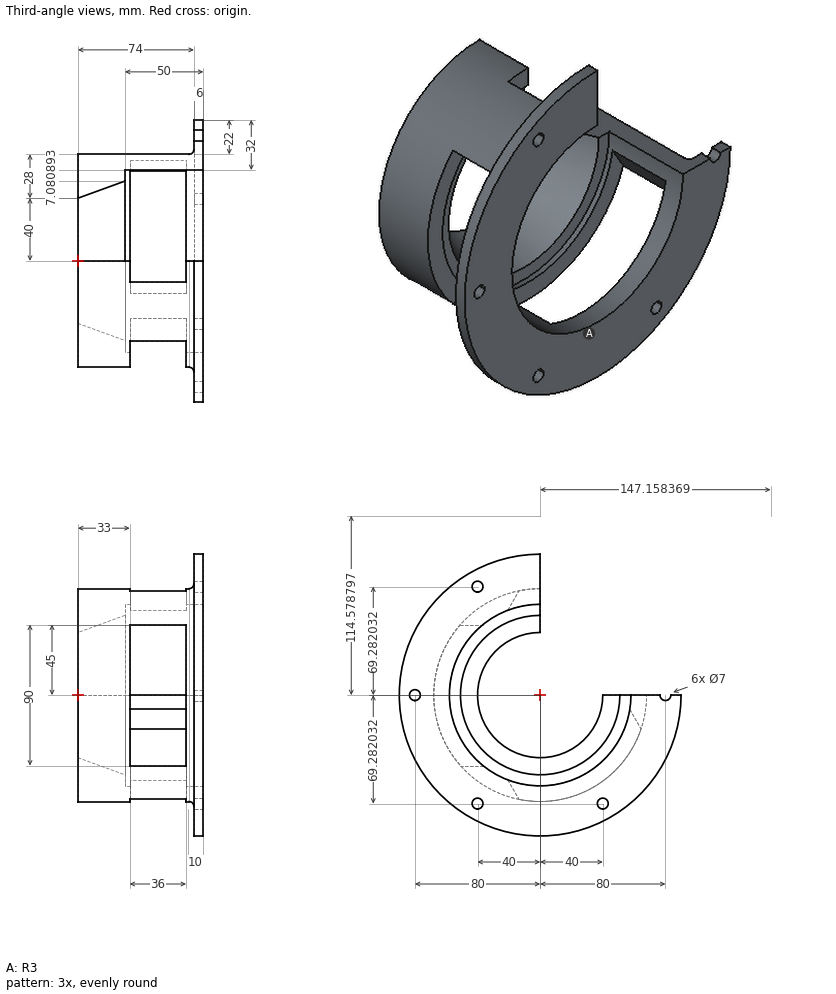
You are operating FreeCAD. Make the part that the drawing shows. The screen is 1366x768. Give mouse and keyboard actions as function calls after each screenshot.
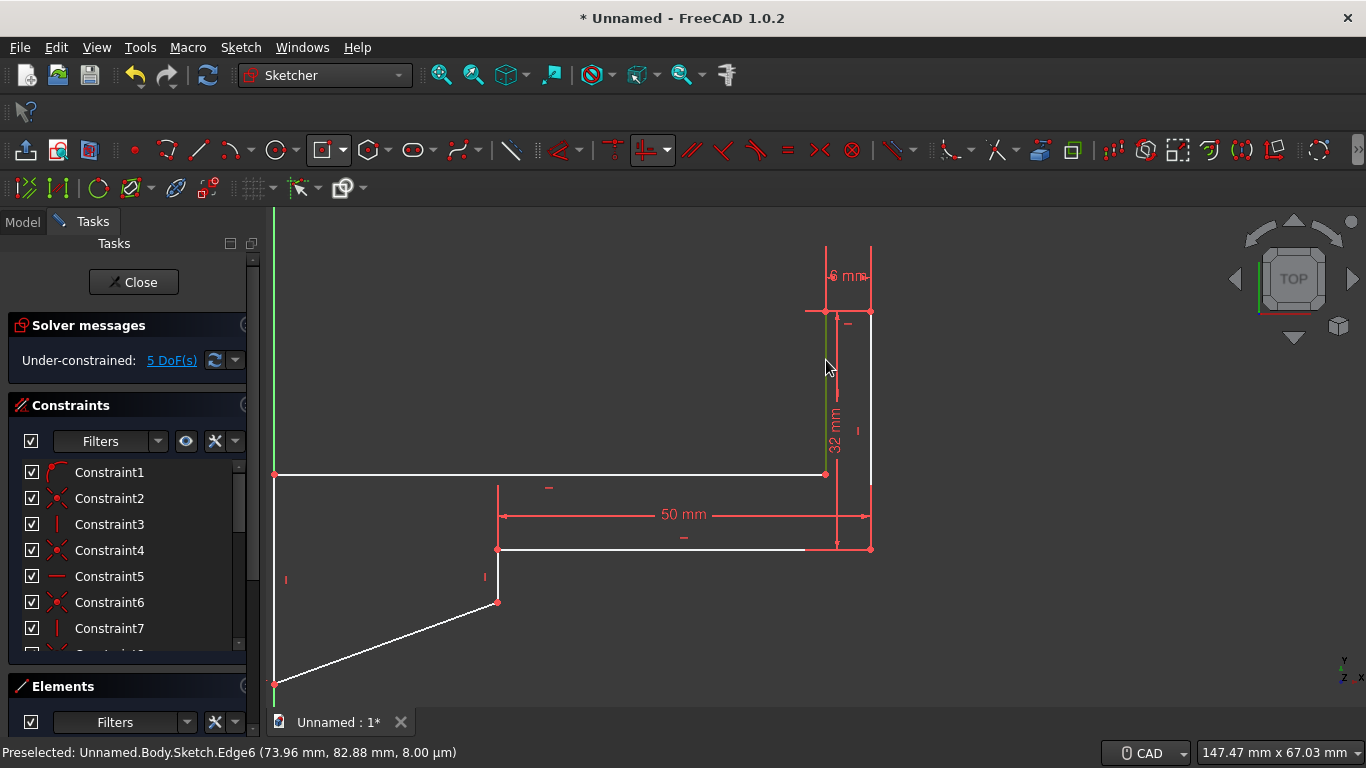
key(i)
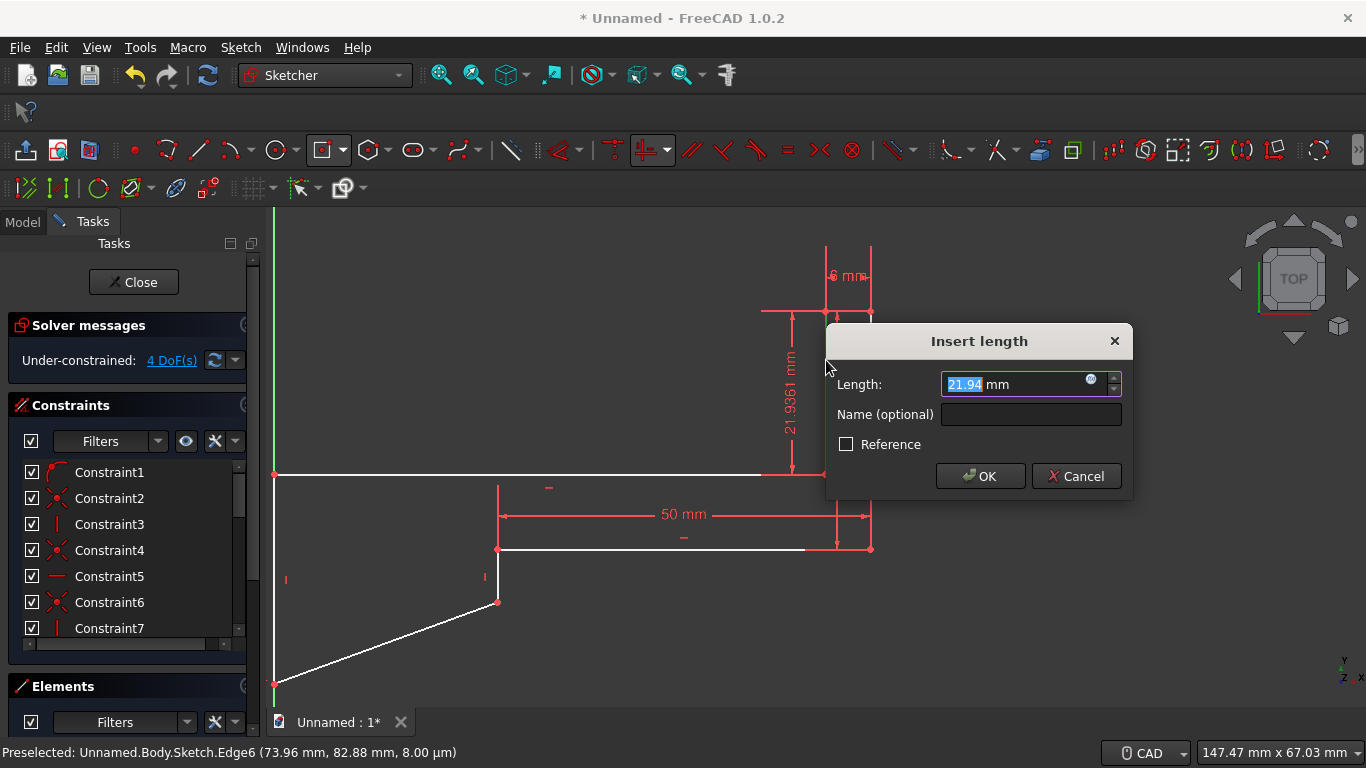
text(22)
key(Return)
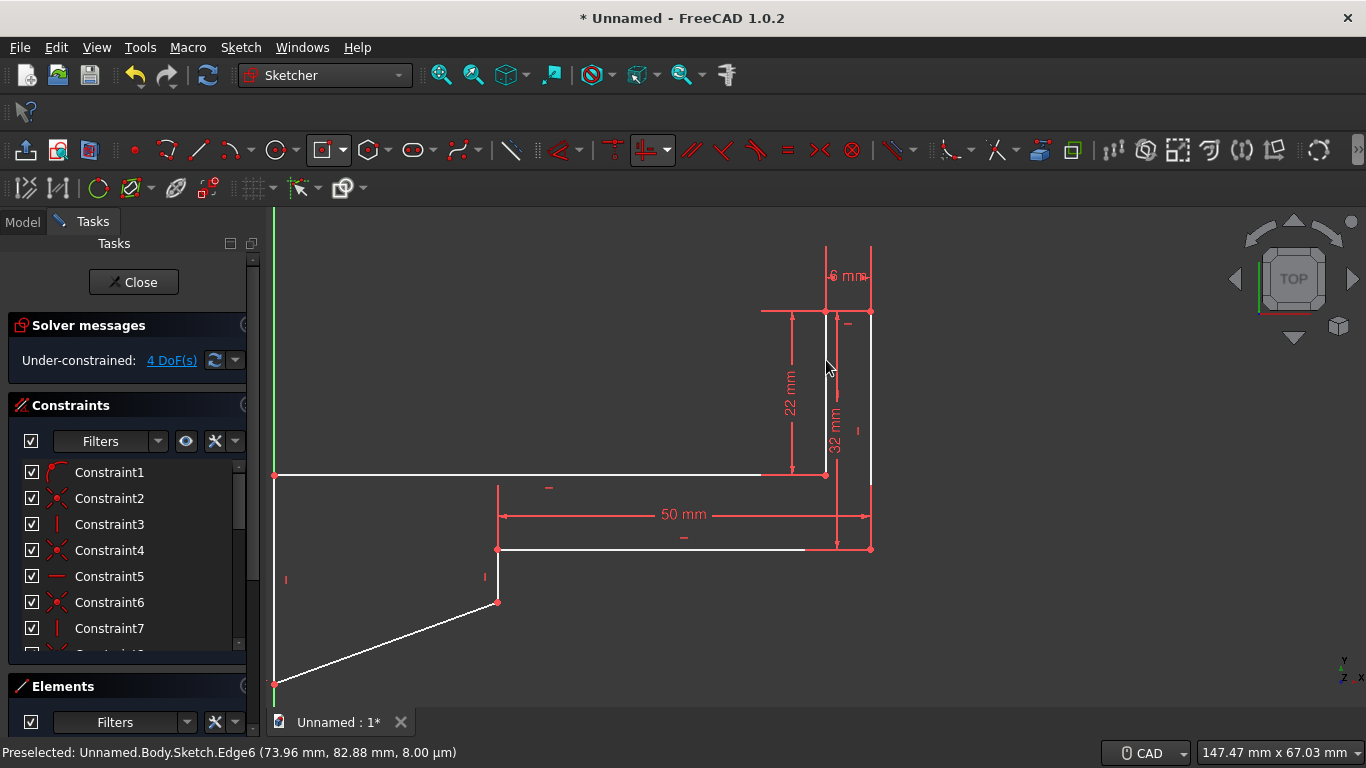
click(660, 475)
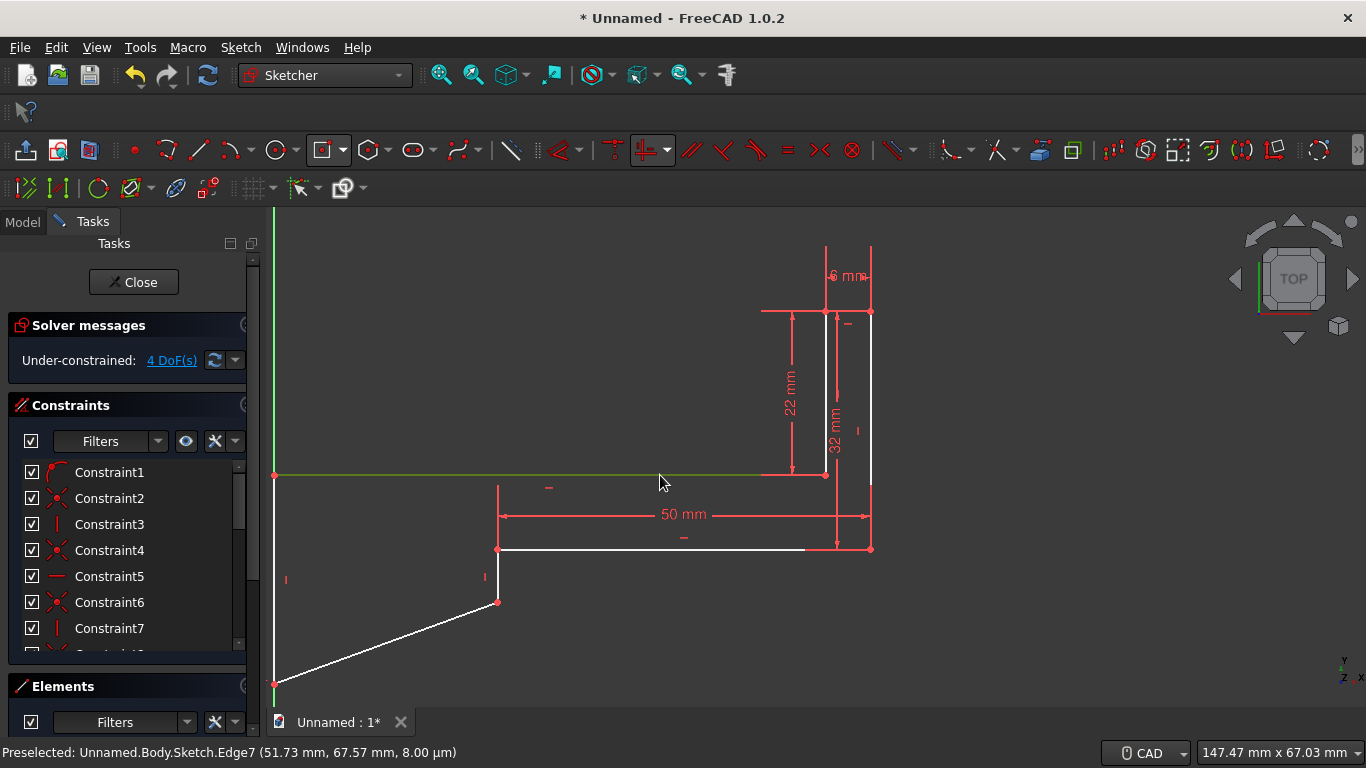
click(582, 150)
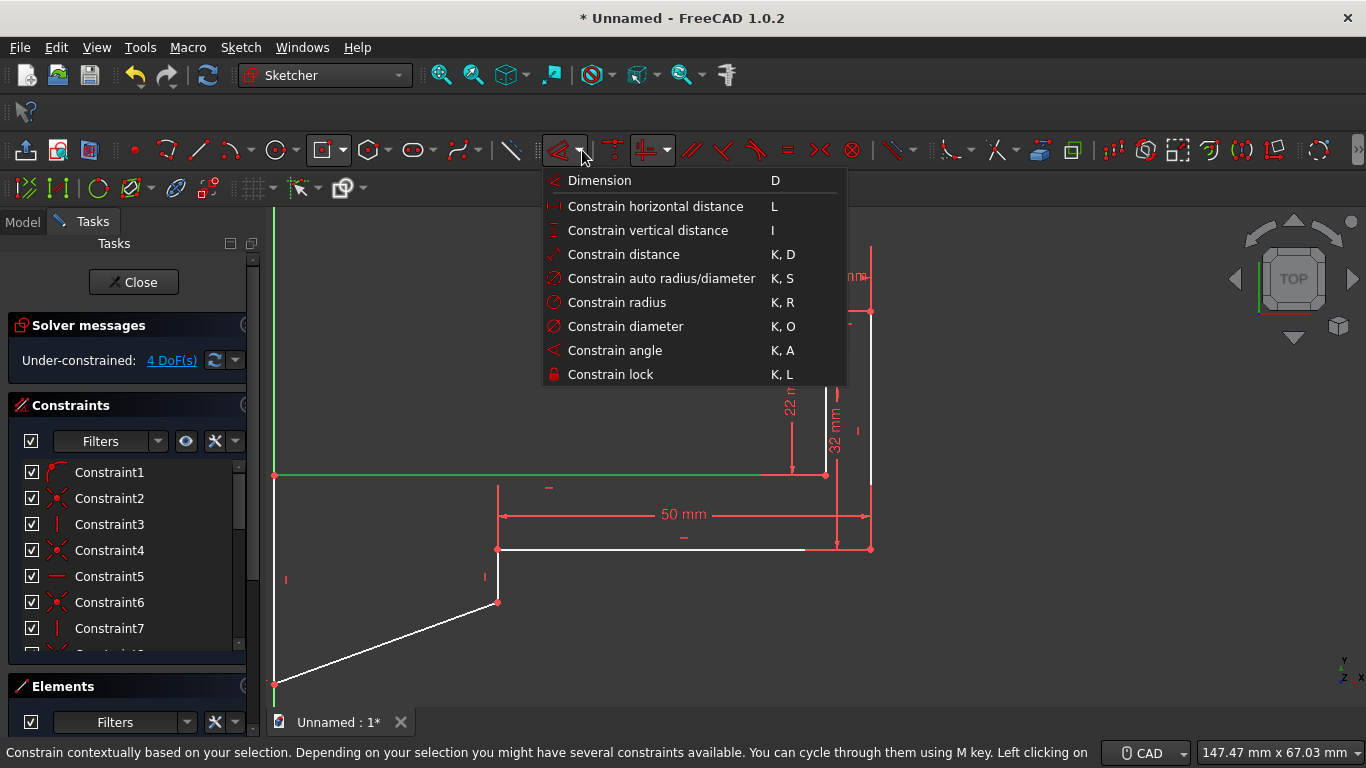
click(695, 206)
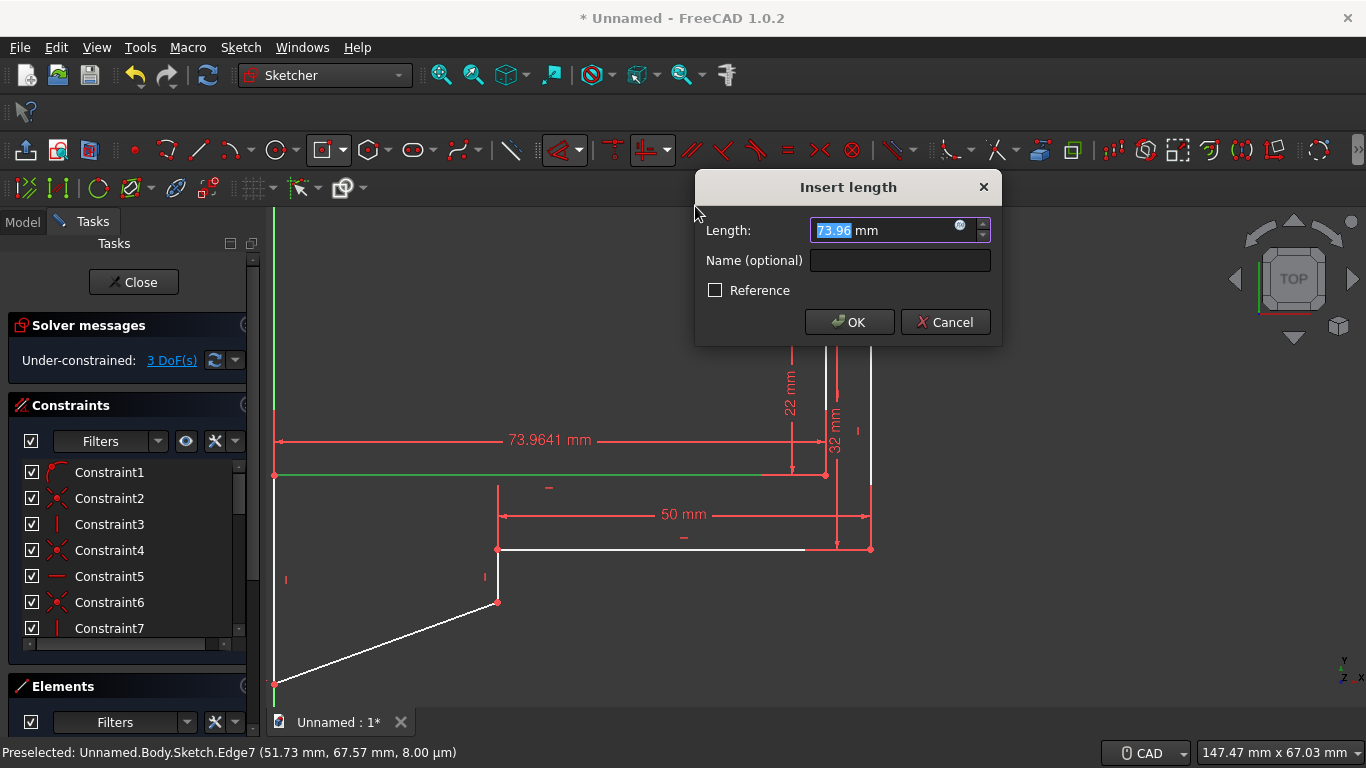
text(74)
key(Return)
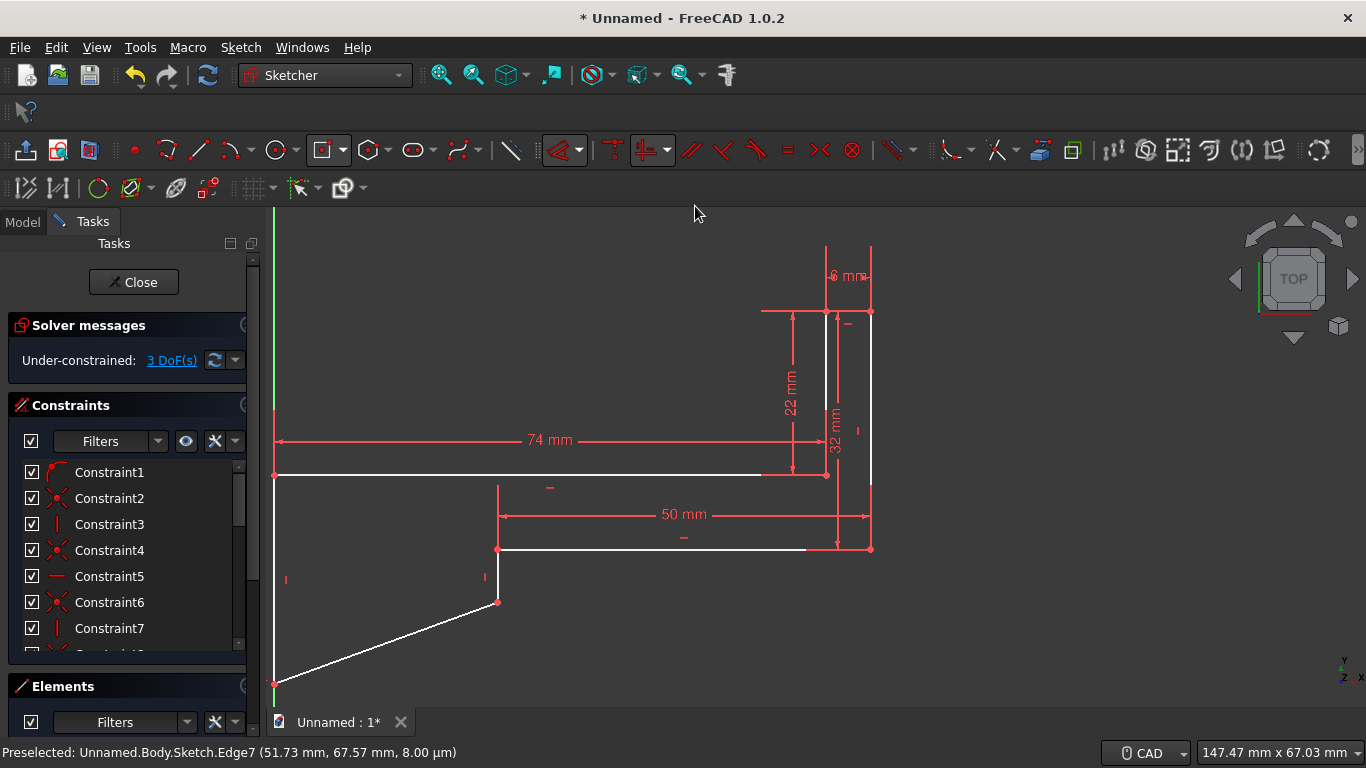
scroll(890, 305, down, 4)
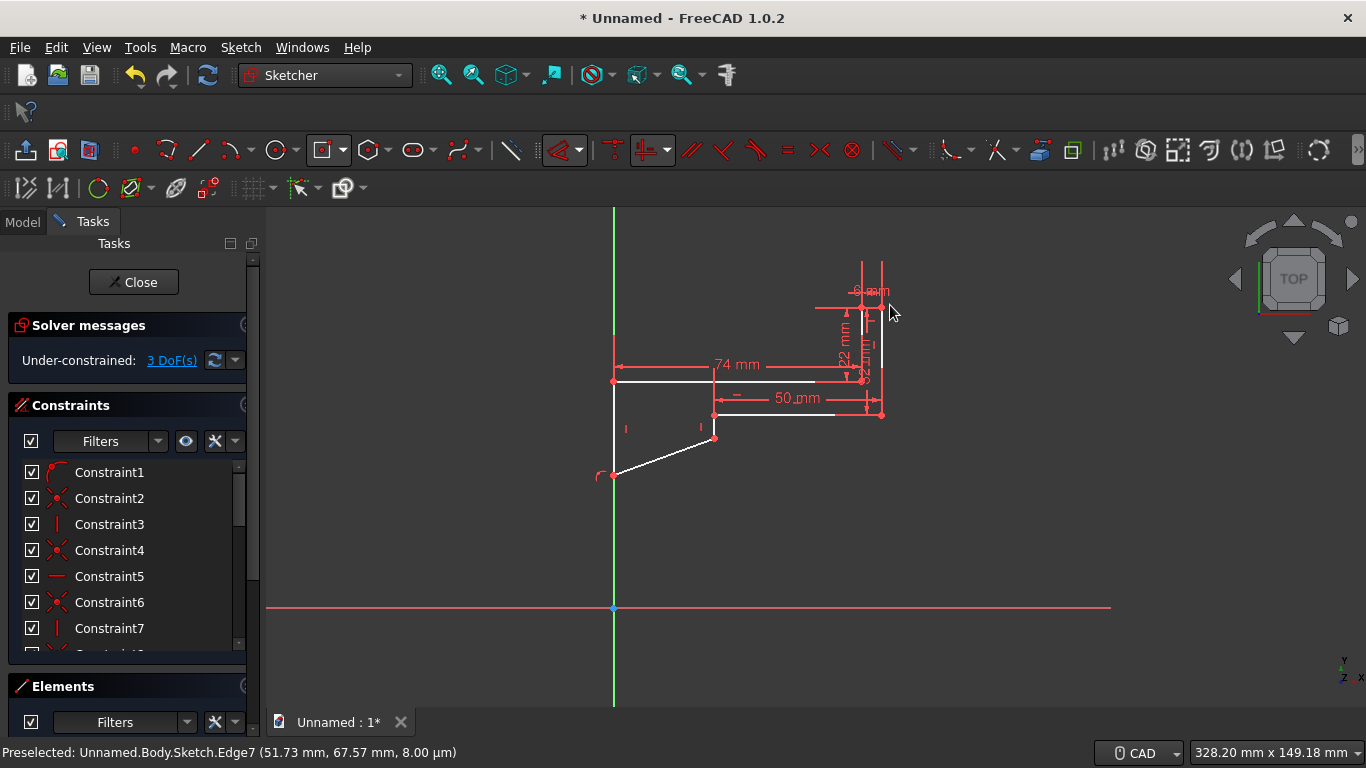
click(614, 410)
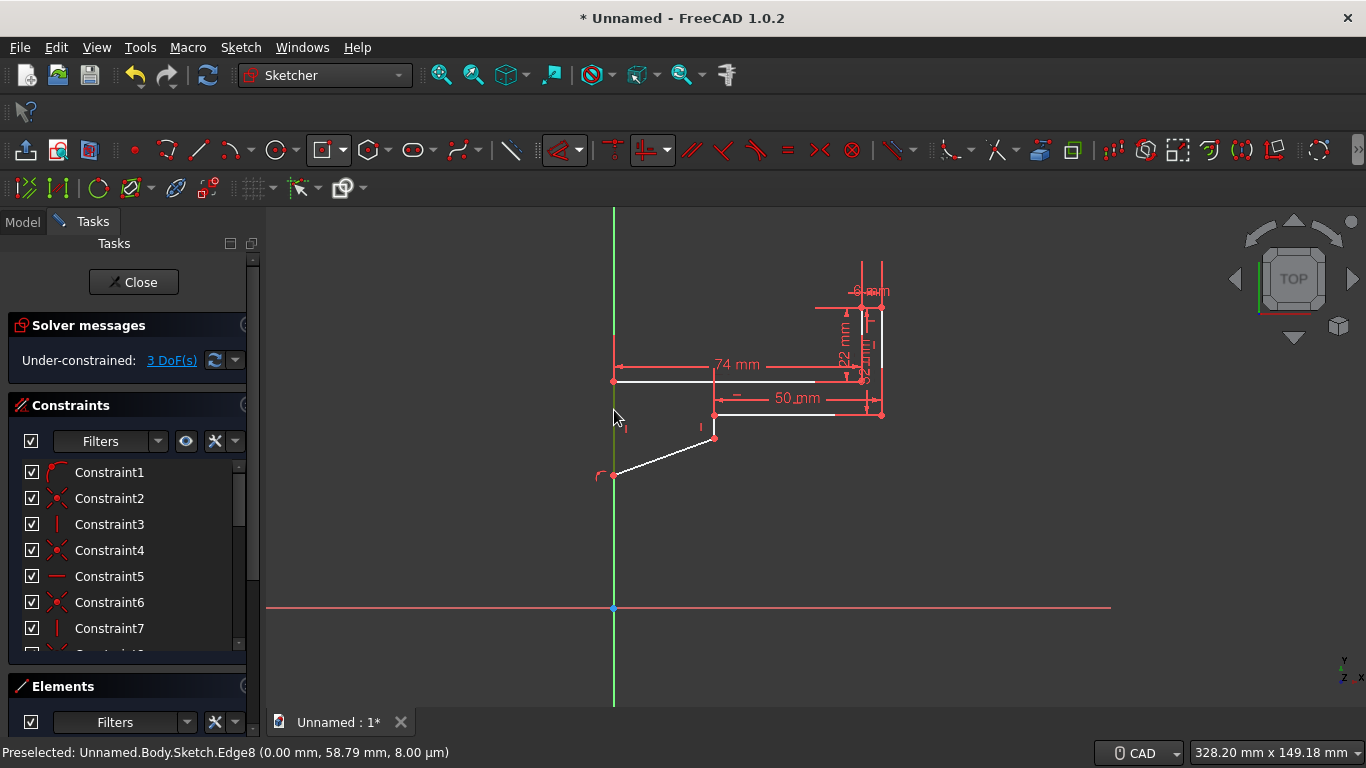
click(582, 150)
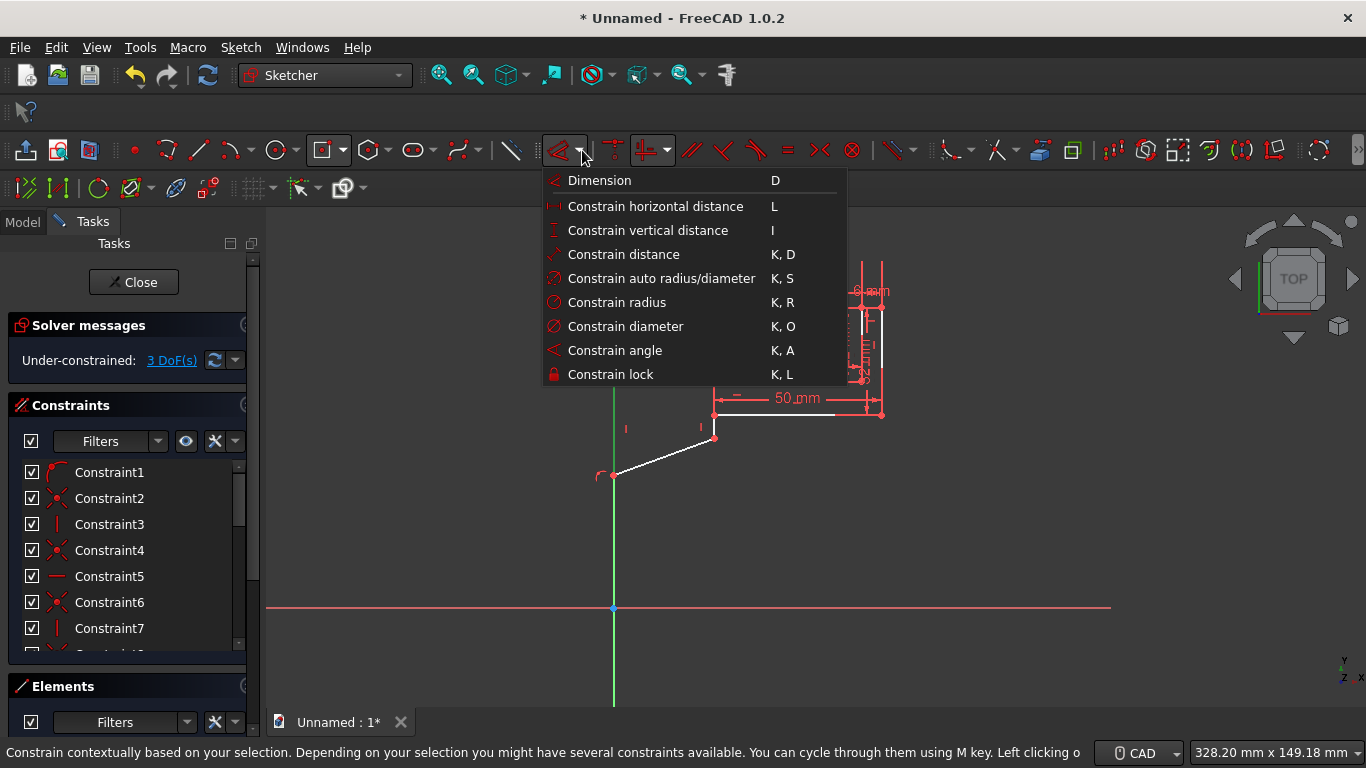
click(695, 230)